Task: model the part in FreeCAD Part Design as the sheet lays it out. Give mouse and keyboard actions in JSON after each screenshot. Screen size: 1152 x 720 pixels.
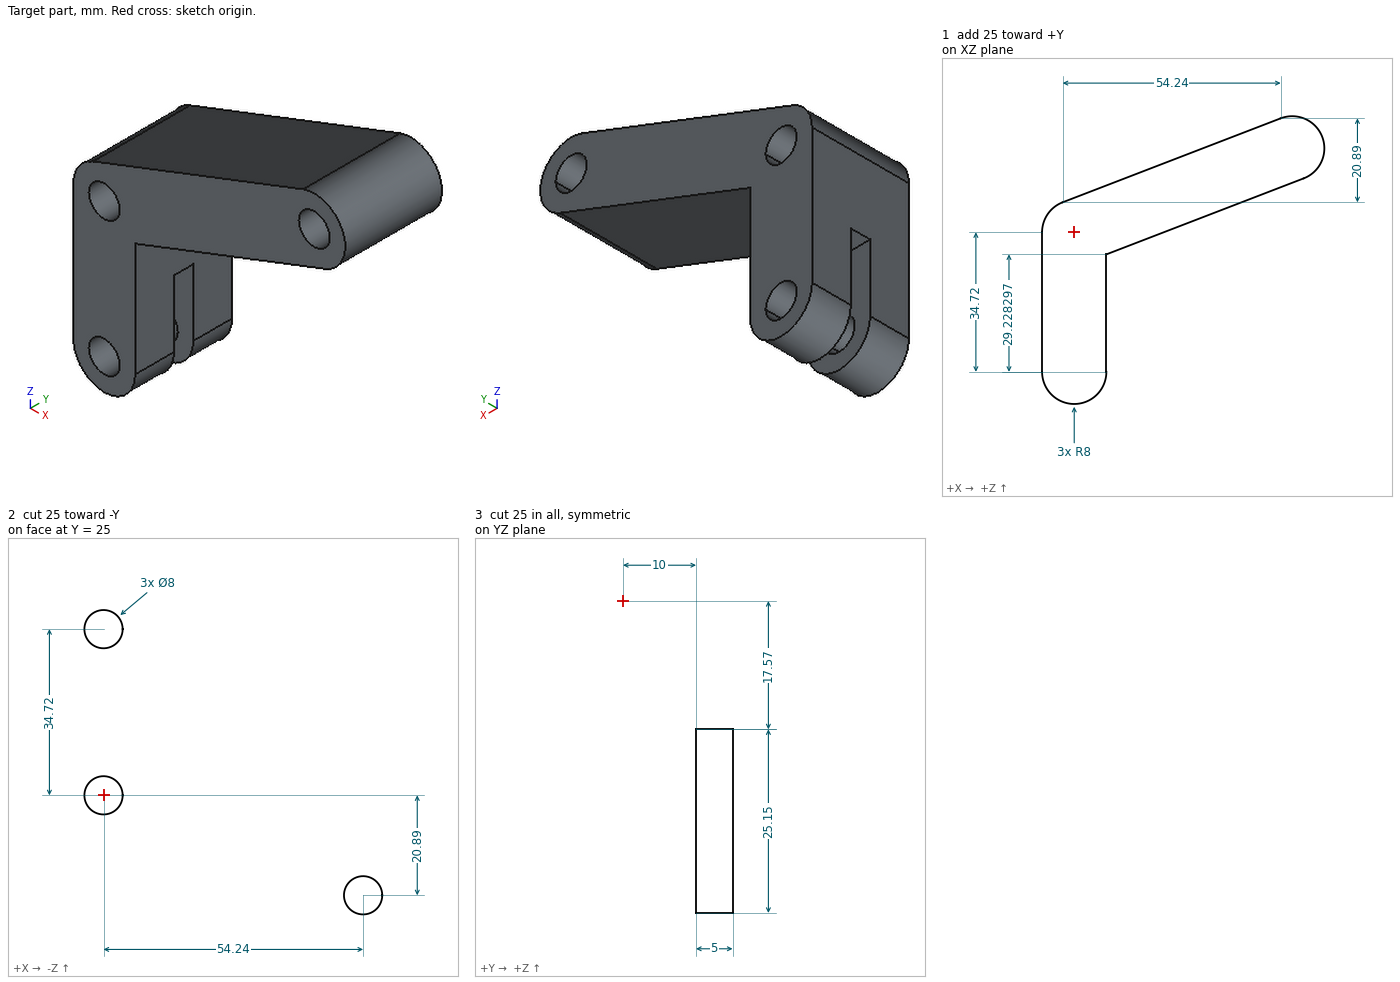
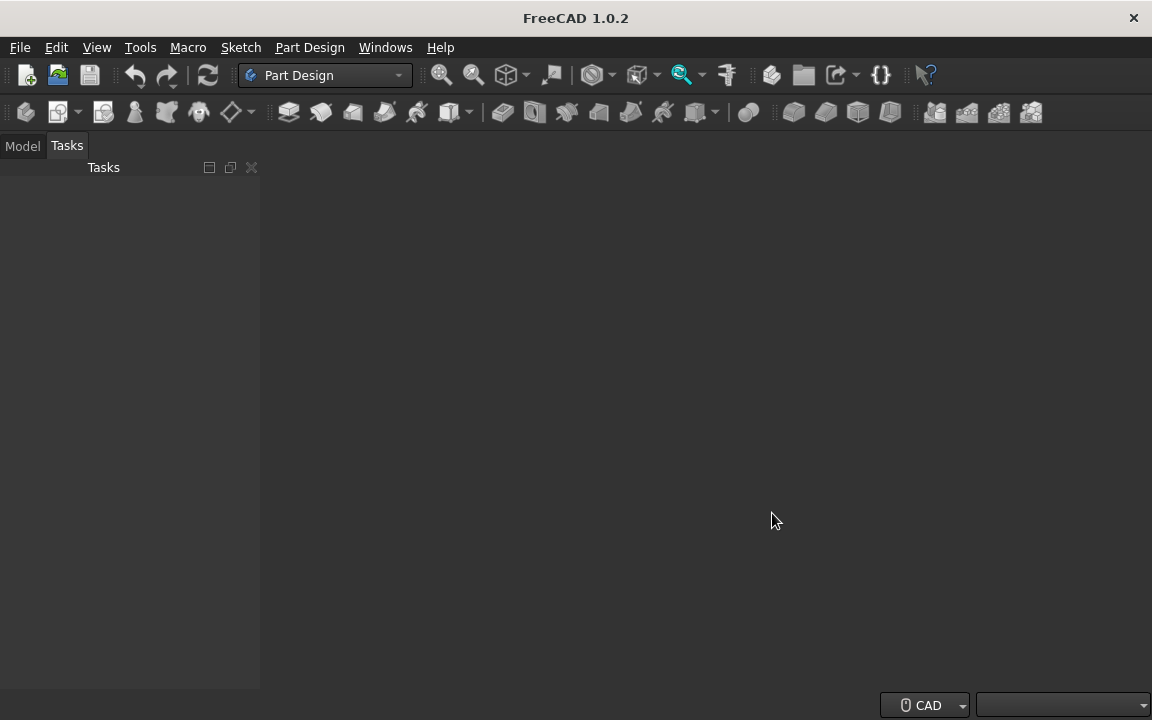
{"action": "left_click", "coordinate": [26, 76]}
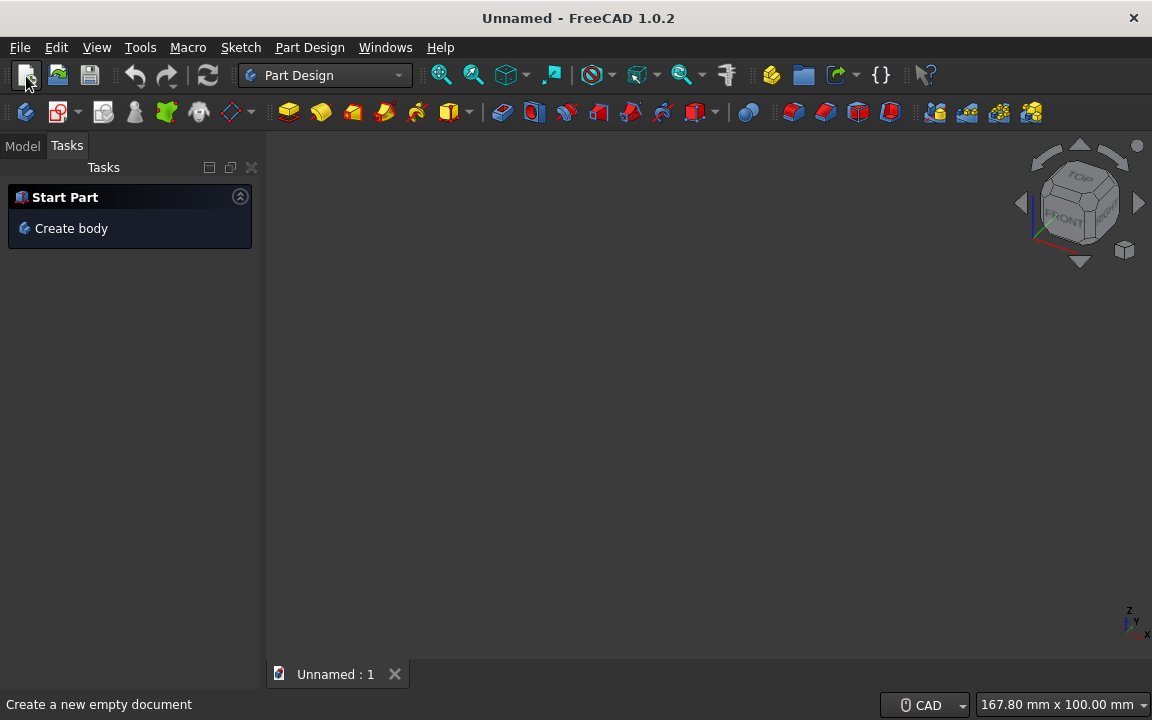
{"action": "left_click", "coordinate": [58, 112]}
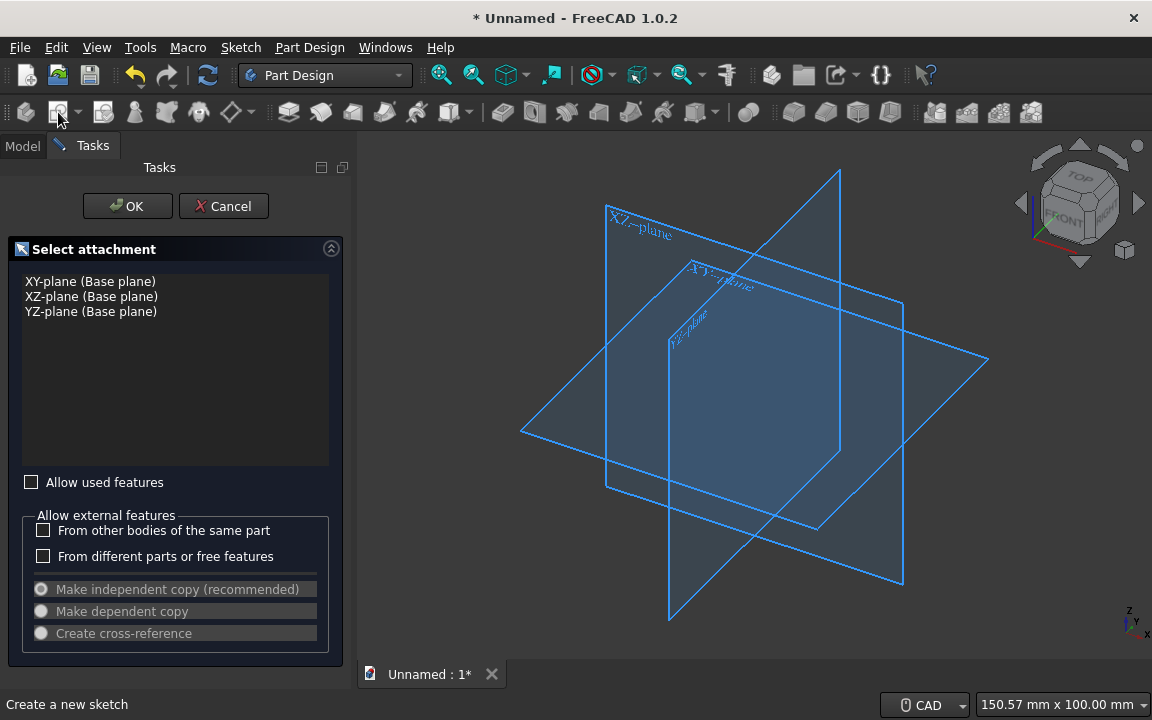
{"action": "left_click", "coordinate": [82, 296]}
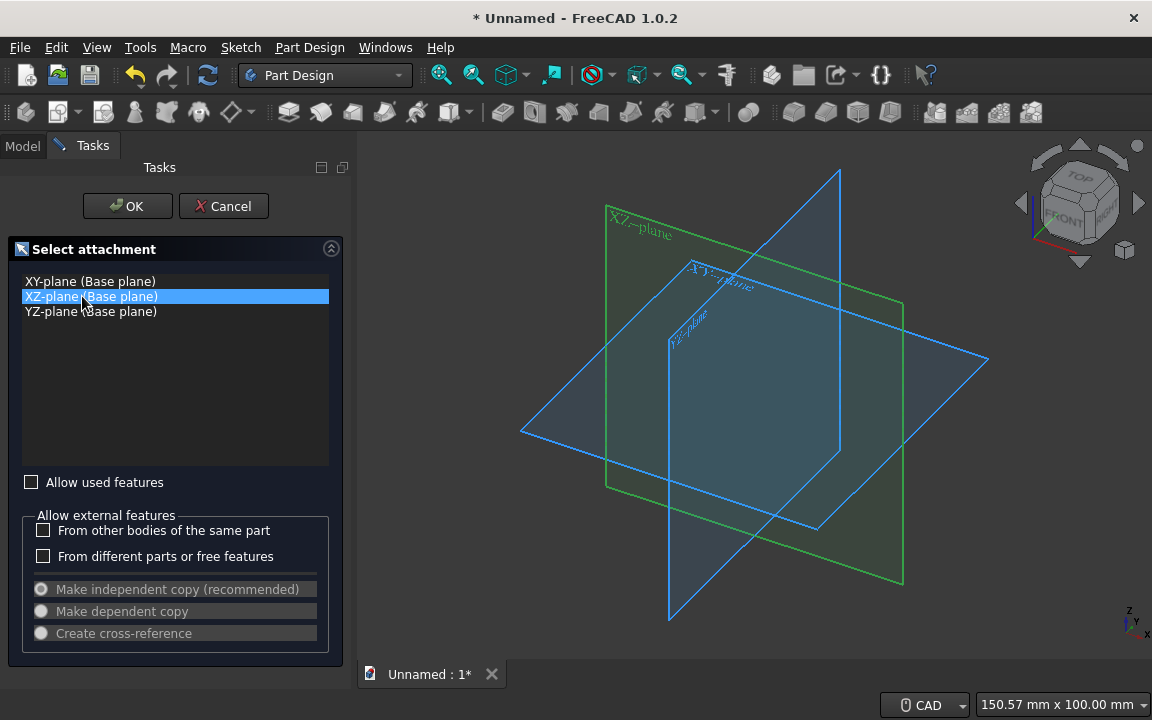
{"action": "left_click", "coordinate": [128, 206]}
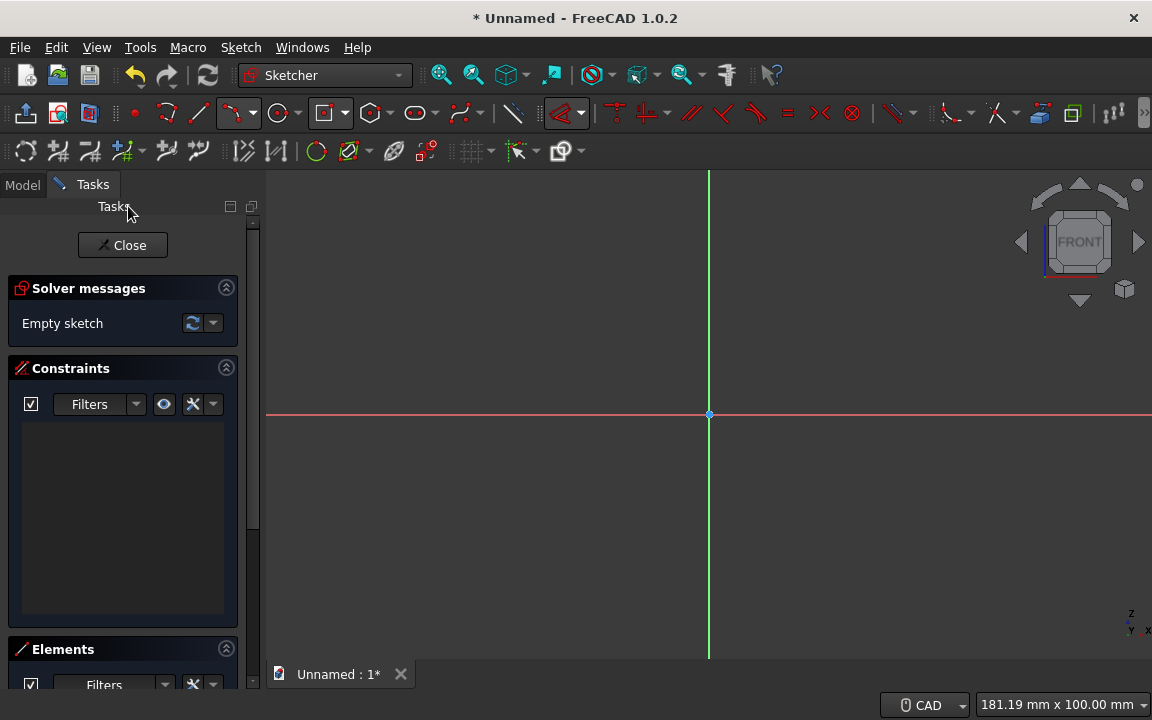
{"action": "scroll", "coordinate": [294, 256], "scroll_direction": "down", "scroll_amount": 1}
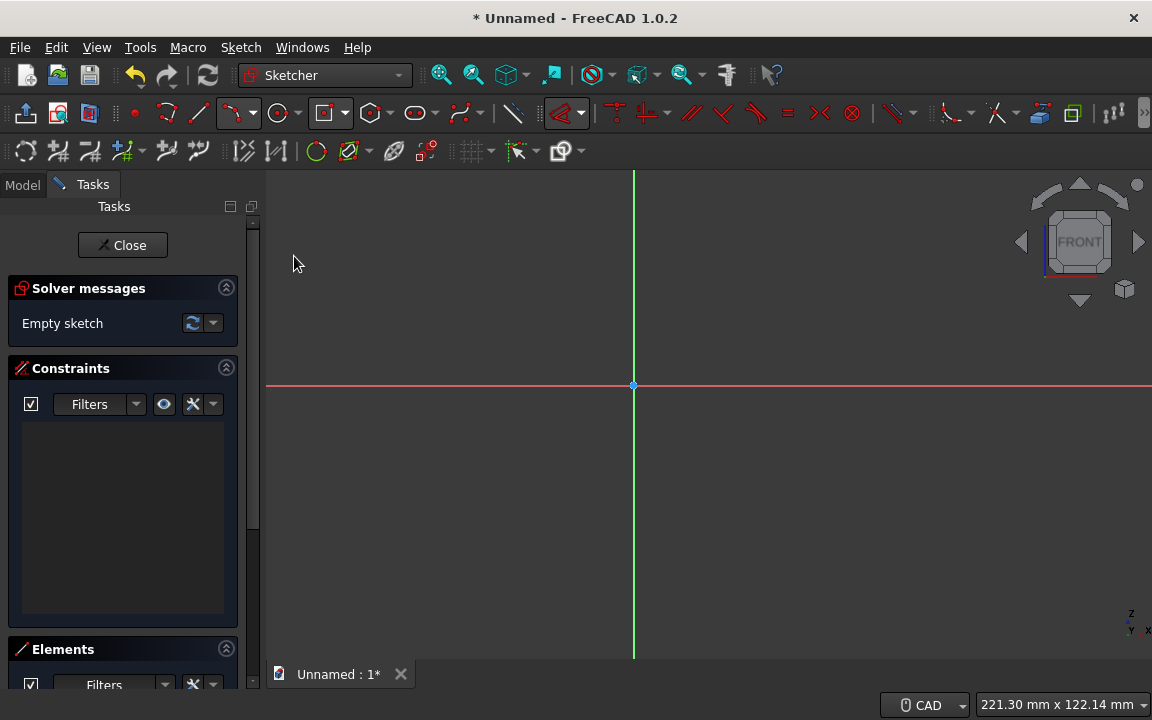
{"action": "left_click", "coordinate": [200, 114]}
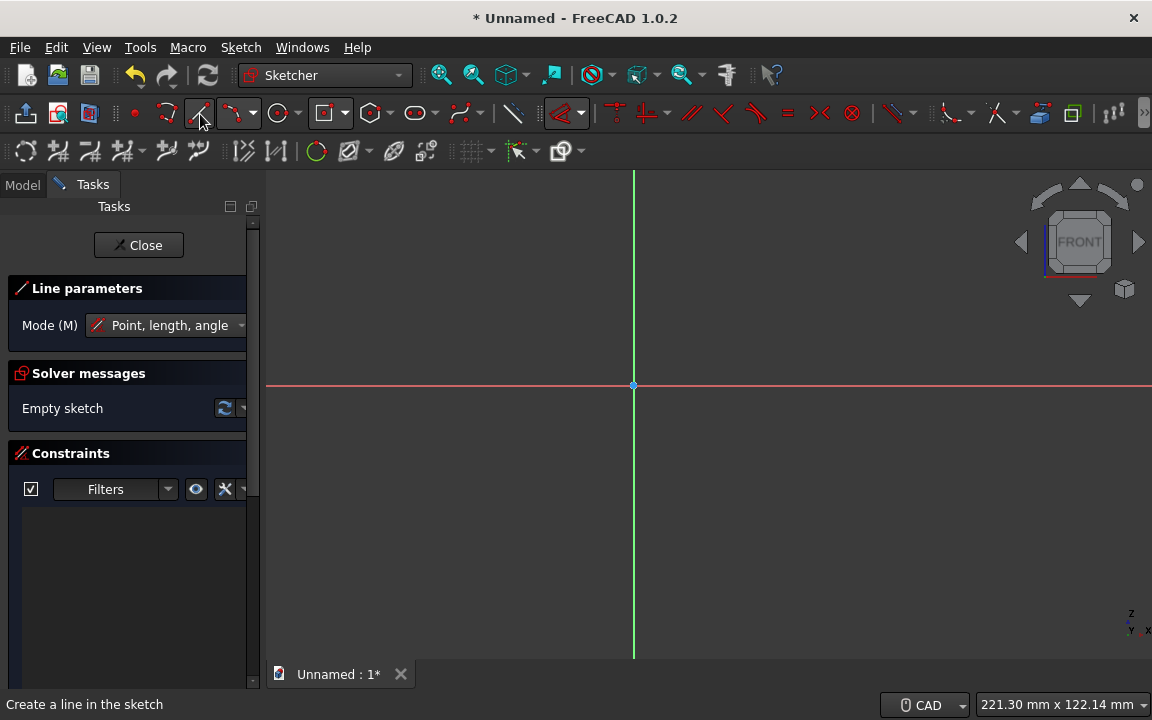
{"action": "left_click", "coordinate": [602, 525]}
{"action": "left_click", "coordinate": [602, 386]}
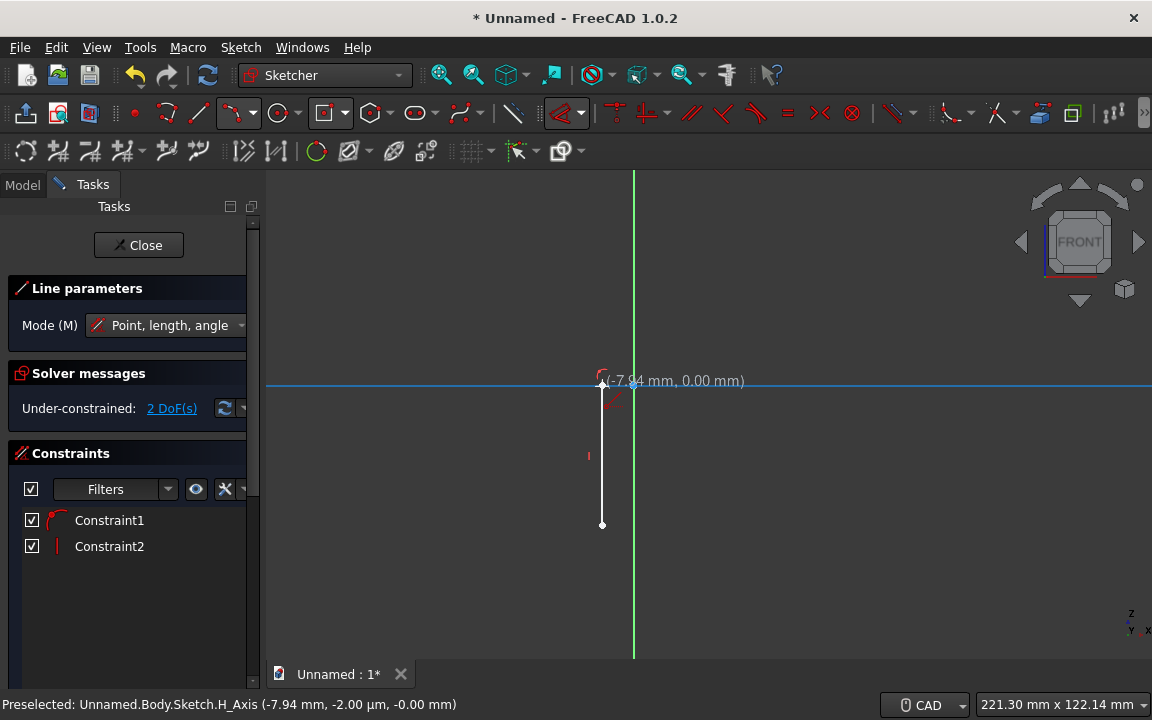
{"action": "scroll", "coordinate": [622, 356], "scroll_direction": "up", "scroll_amount": 2}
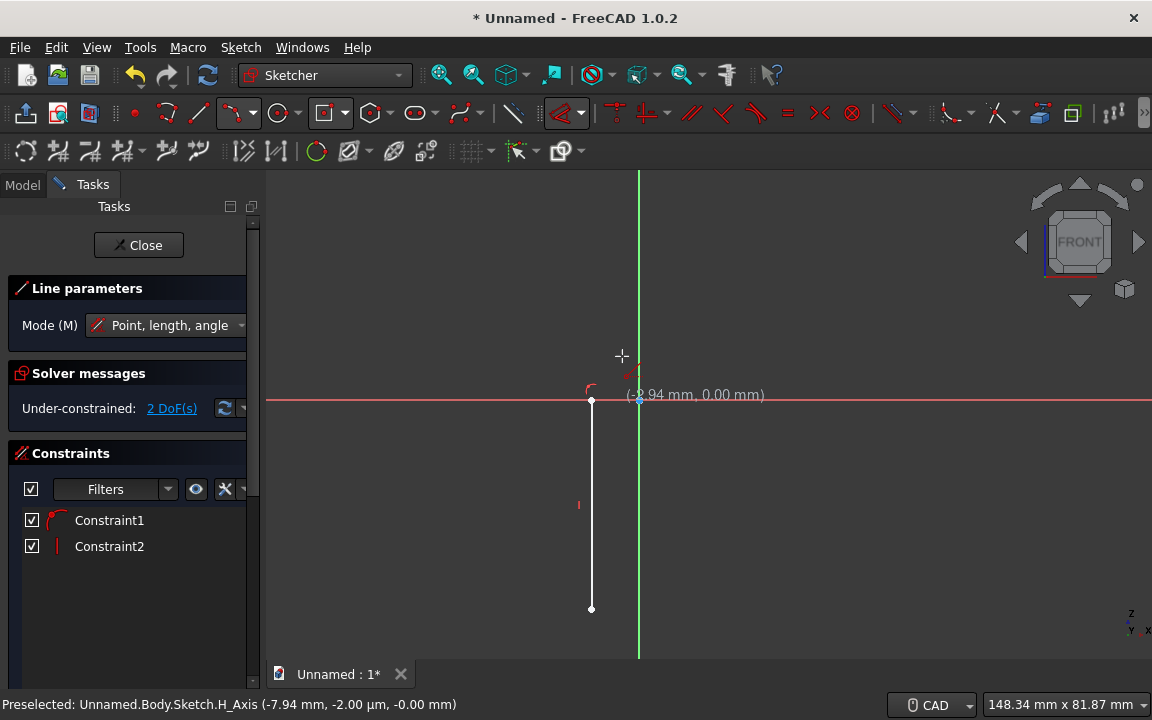
{"action": "left_click", "coordinate": [622, 356]}
{"action": "left_click", "coordinate": [946, 231]}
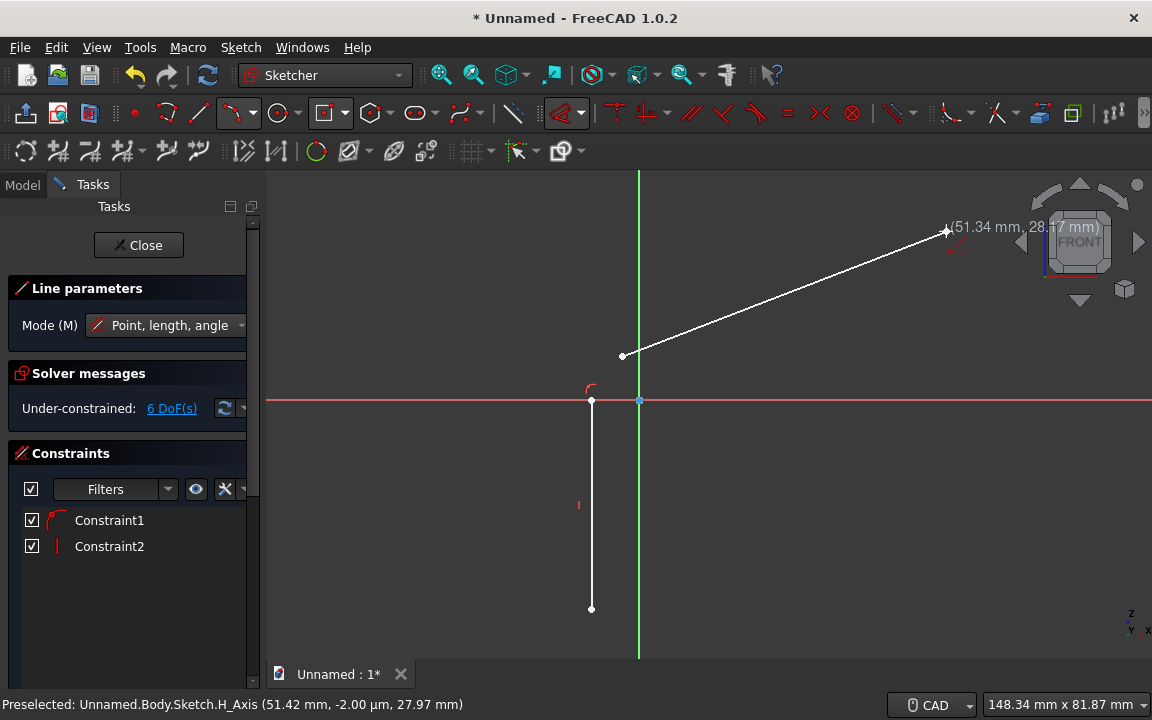
{"action": "left_click", "coordinate": [168, 114]}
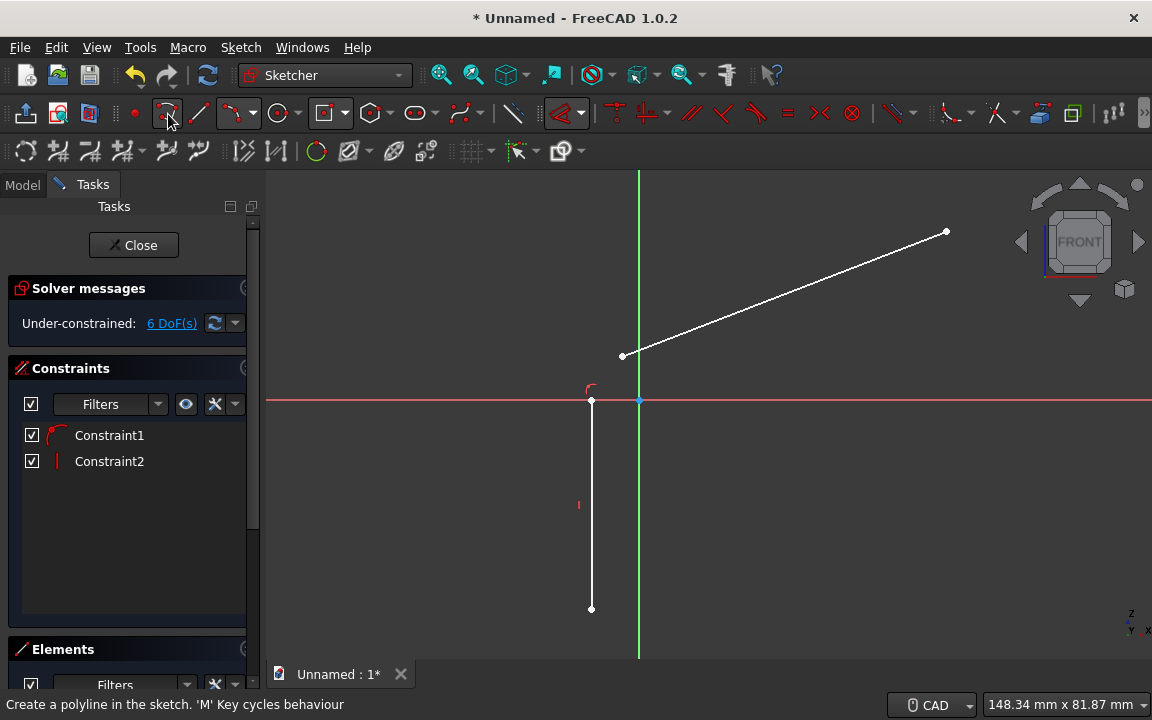
{"action": "left_click", "coordinate": [981, 320]}
{"action": "left_click", "coordinate": [687, 433]}
{"action": "left_click", "coordinate": [687, 608]}
{"action": "right_click", "coordinate": [687, 608]}